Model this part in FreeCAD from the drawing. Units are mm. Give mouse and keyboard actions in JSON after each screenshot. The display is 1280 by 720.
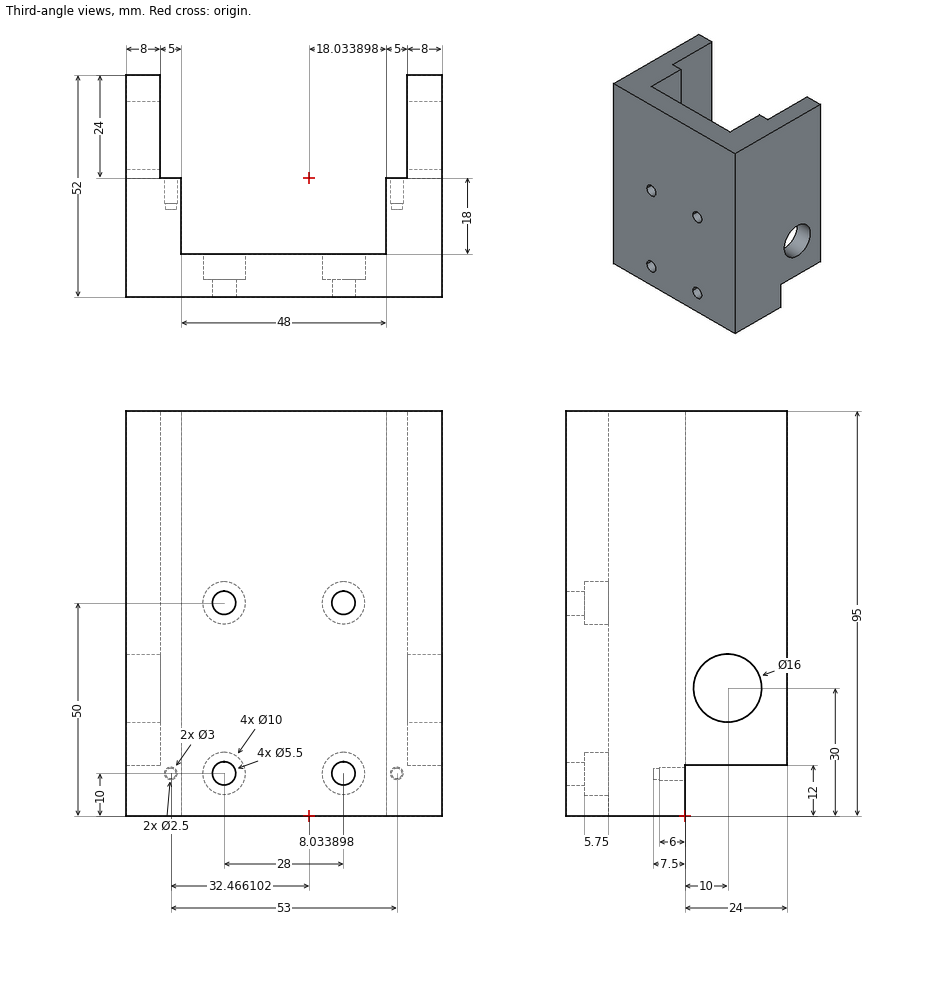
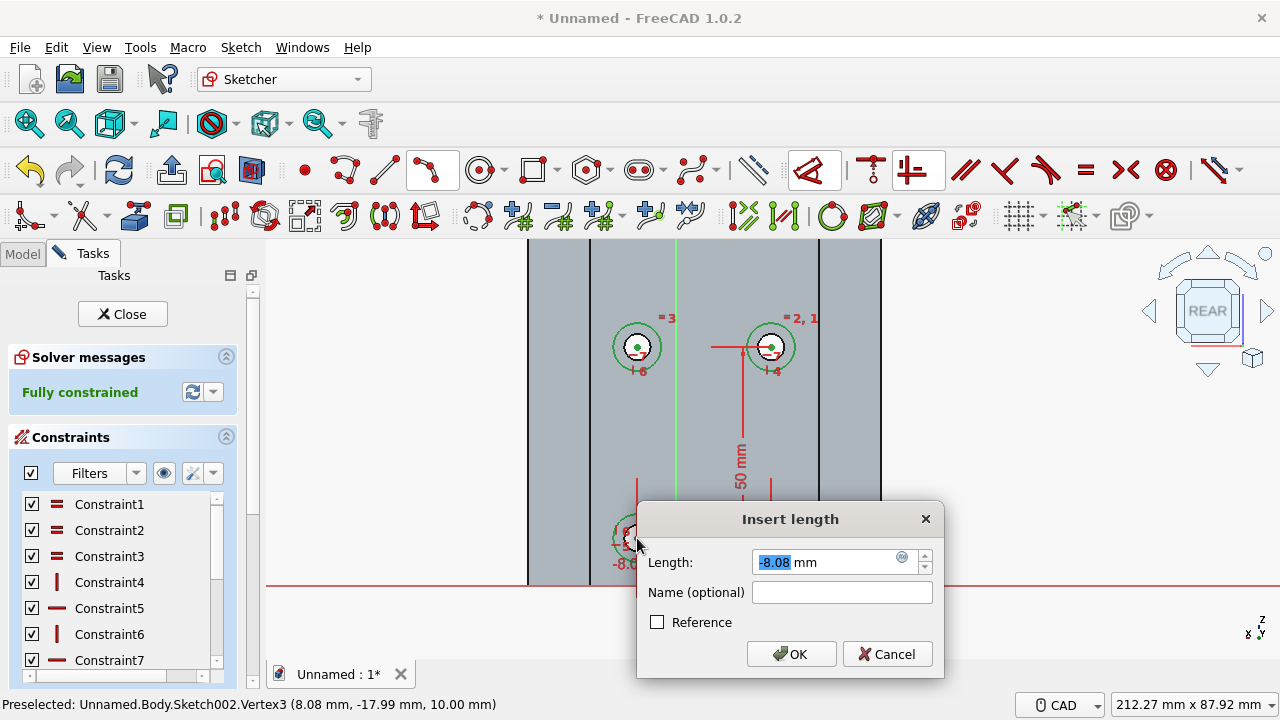
{"action": "type", "text": "-8.033898"}
{"action": "key", "text": "Return"}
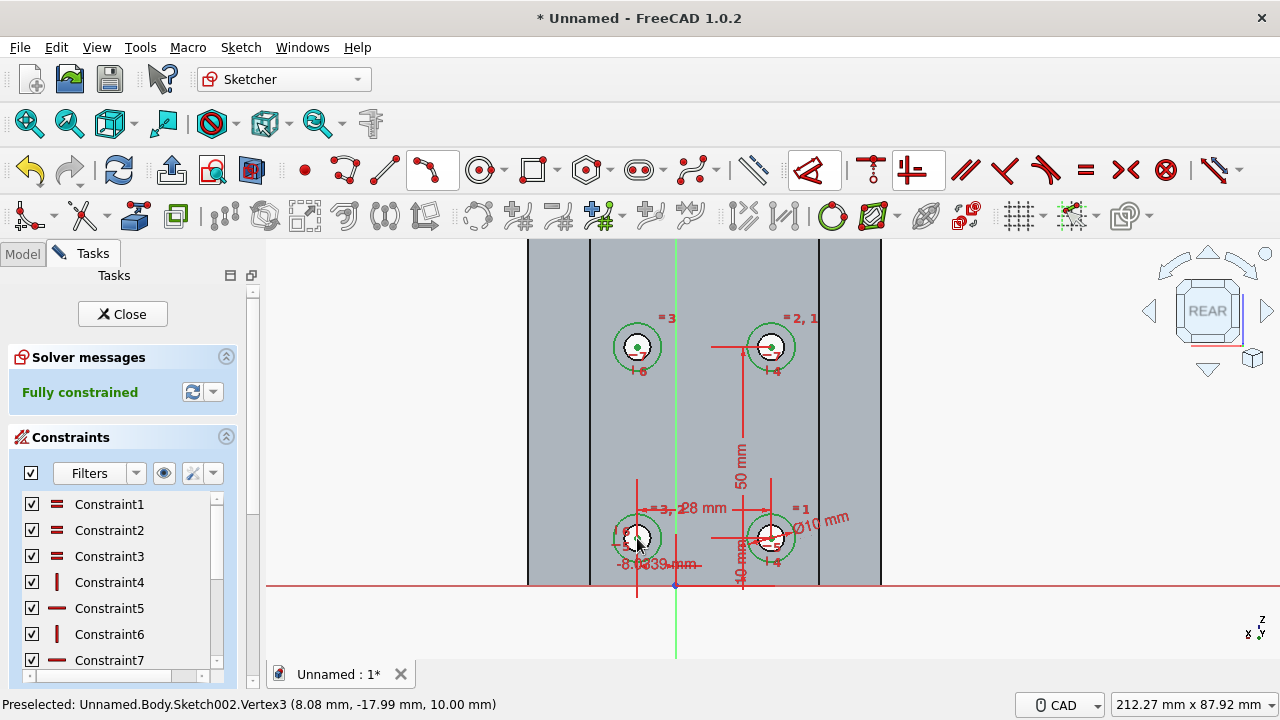
{"action": "left_click", "coordinate": [123, 314]}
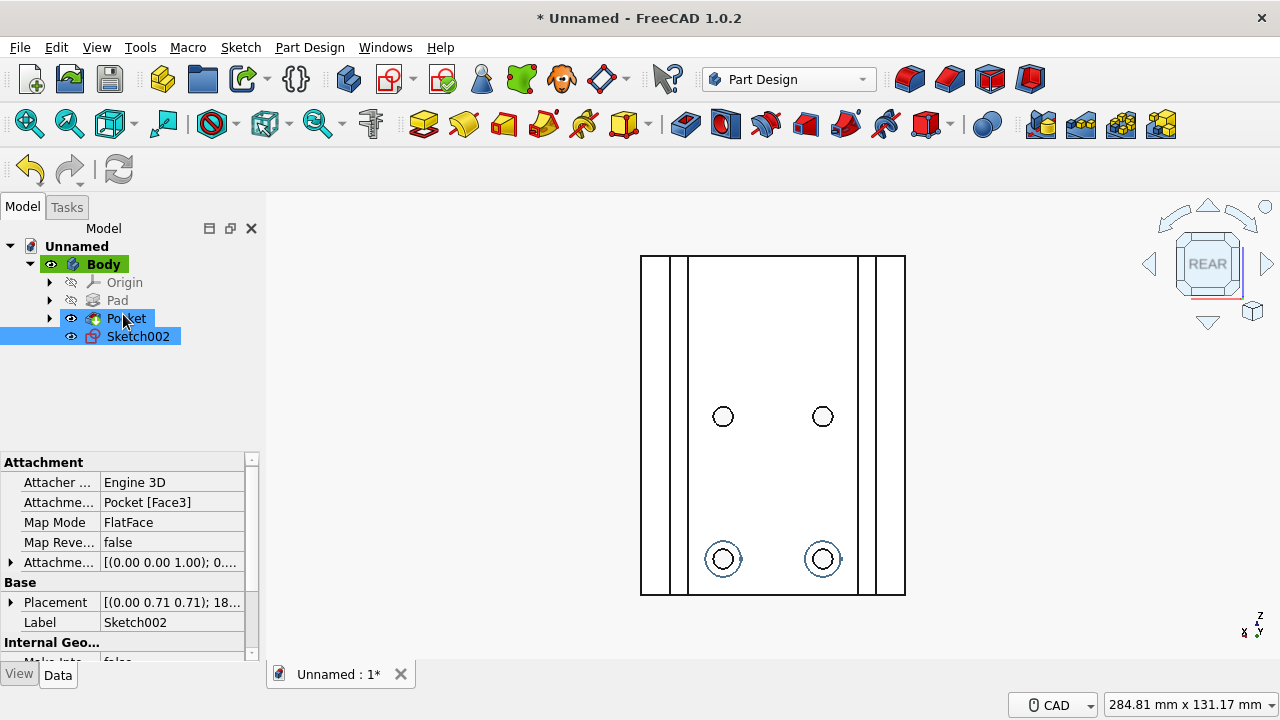
{"action": "left_click", "coordinate": [686, 124]}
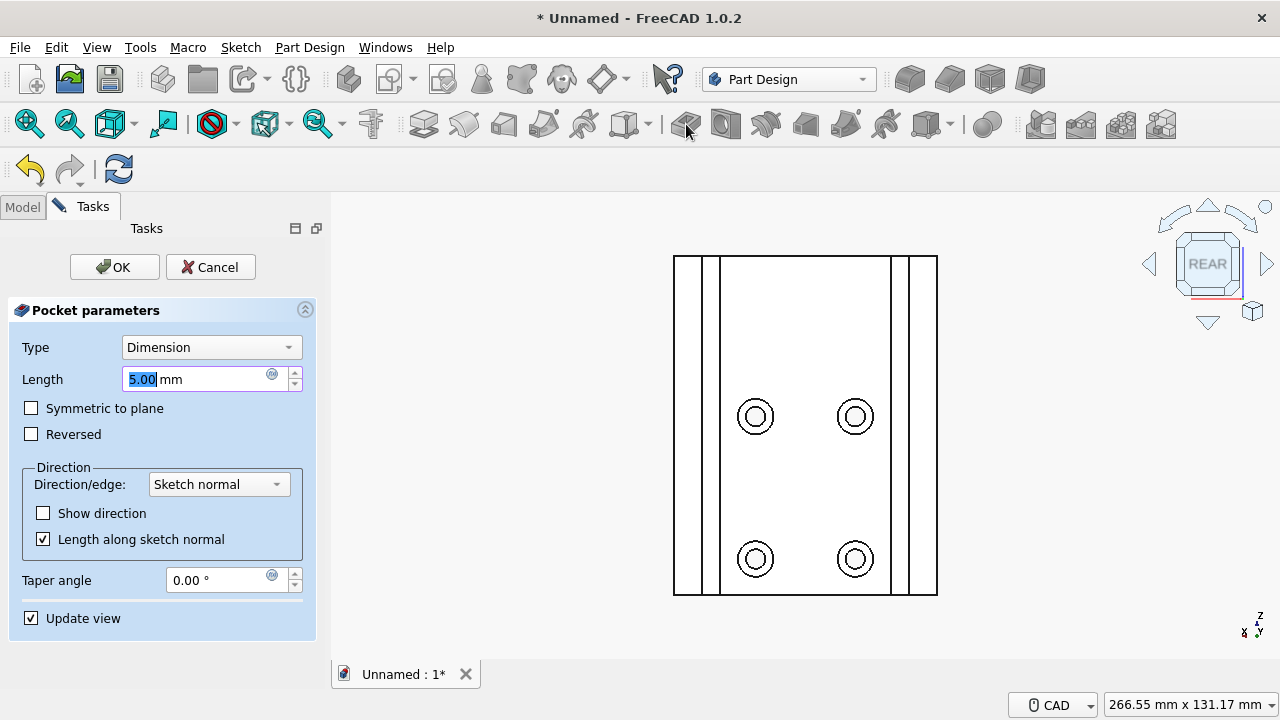
{"action": "type", "text": "5.75"}
{"action": "key", "text": "Tab"}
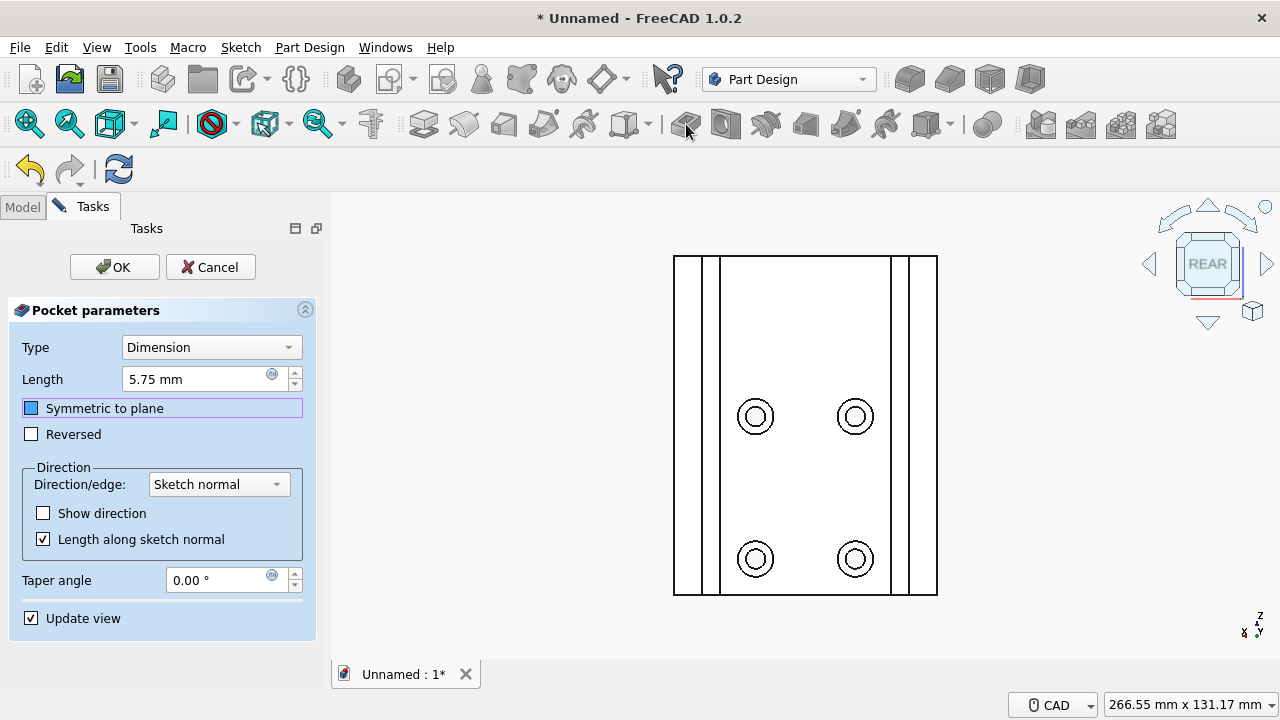
{"action": "left_click", "coordinate": [115, 267]}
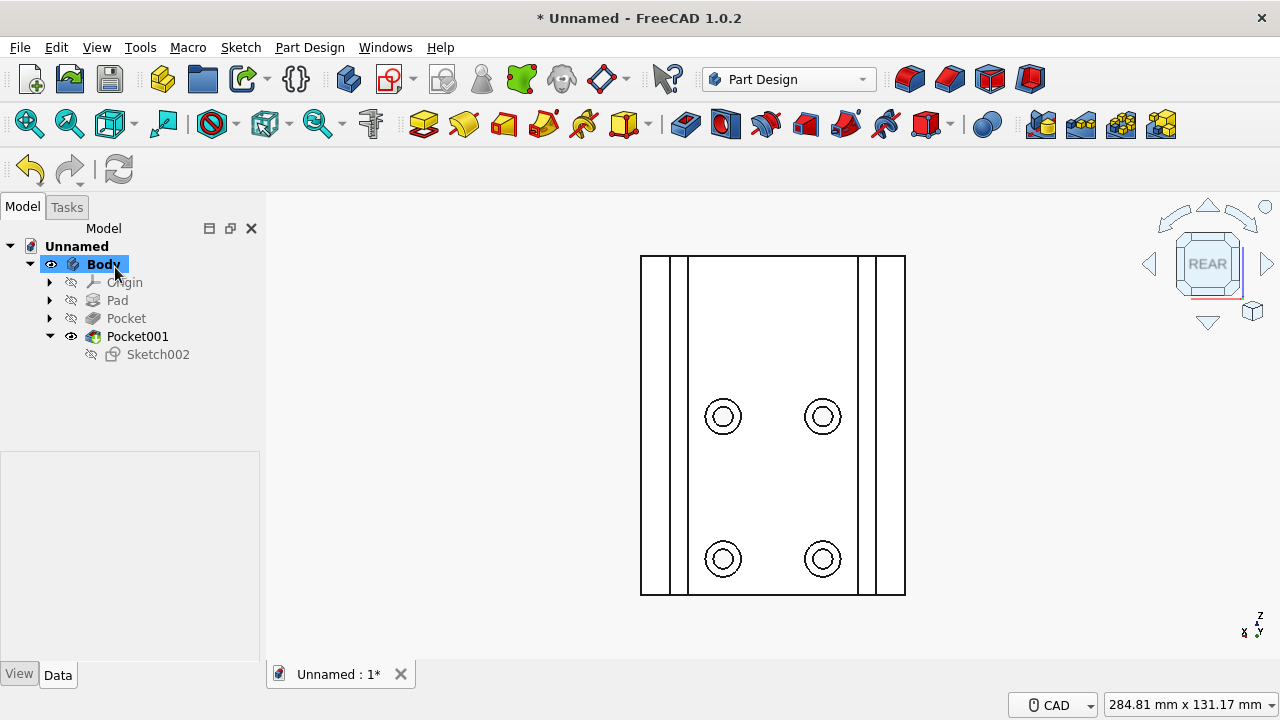
{"action": "key", "text": "6"}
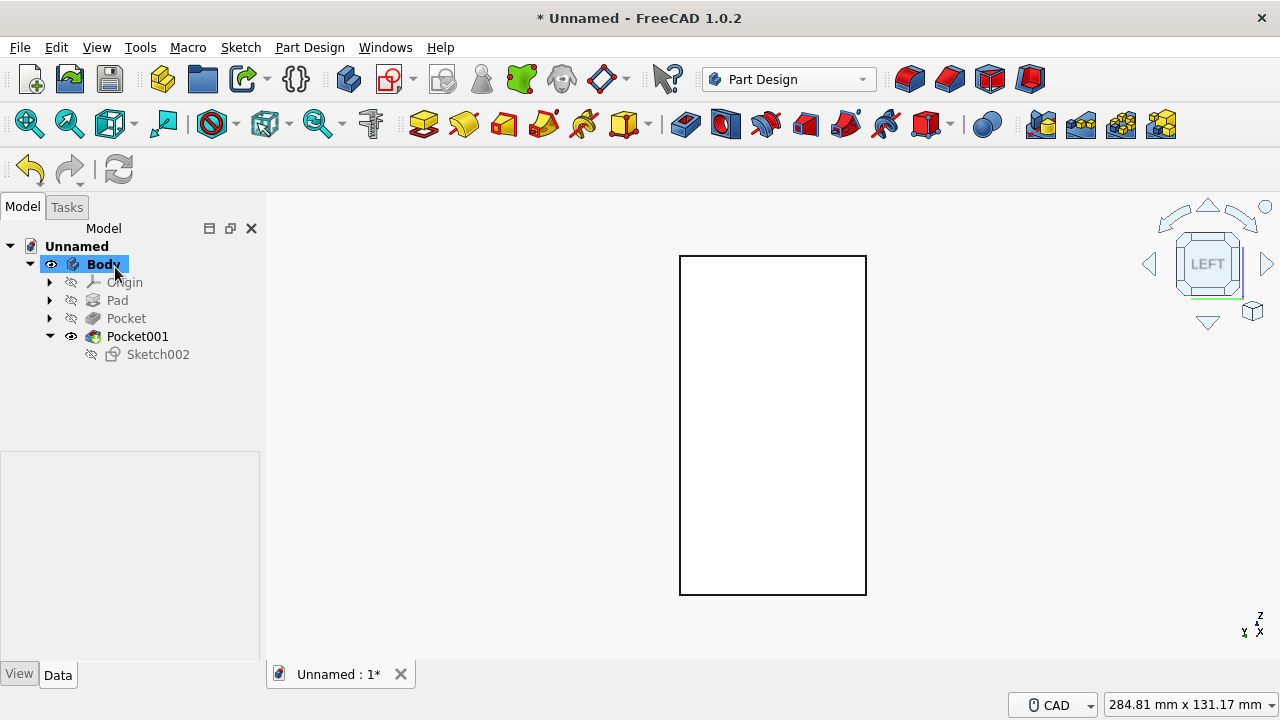
{"action": "left_click", "coordinate": [773, 376]}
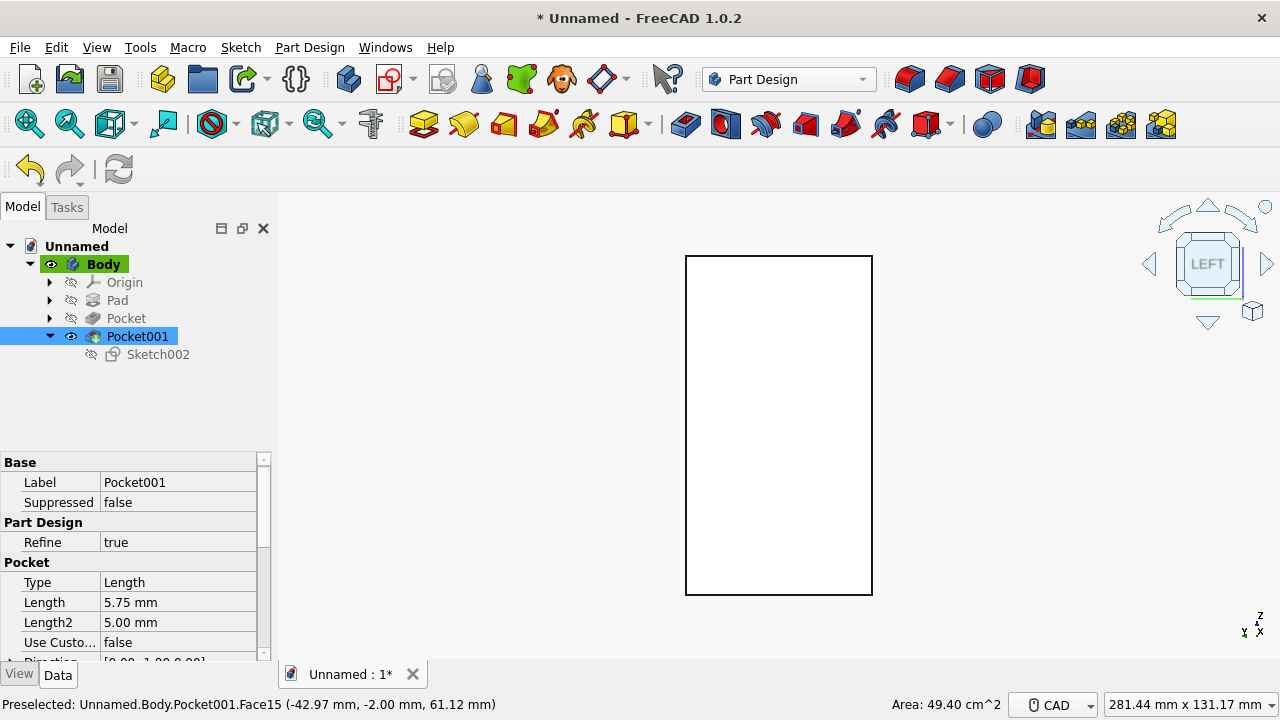
{"action": "left_click", "coordinate": [390, 80]}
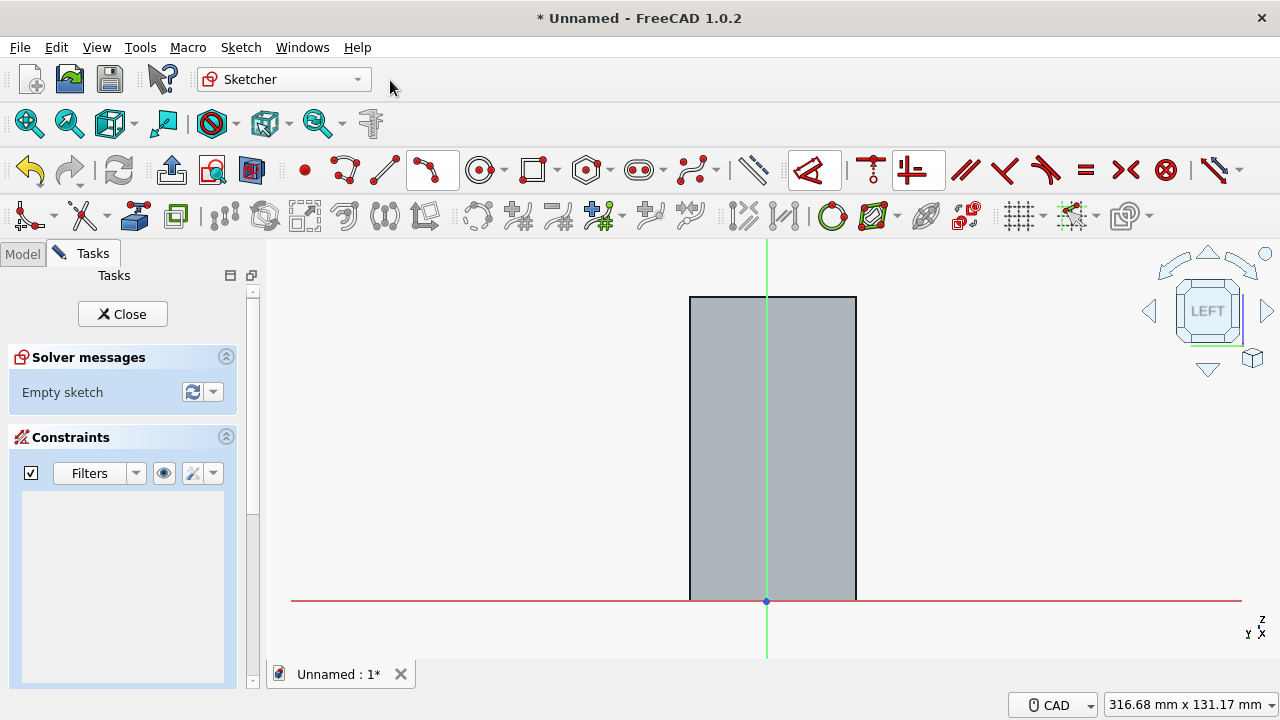
{"action": "scroll", "coordinate": [732, 603], "scroll_direction": "up", "scroll_amount": 10}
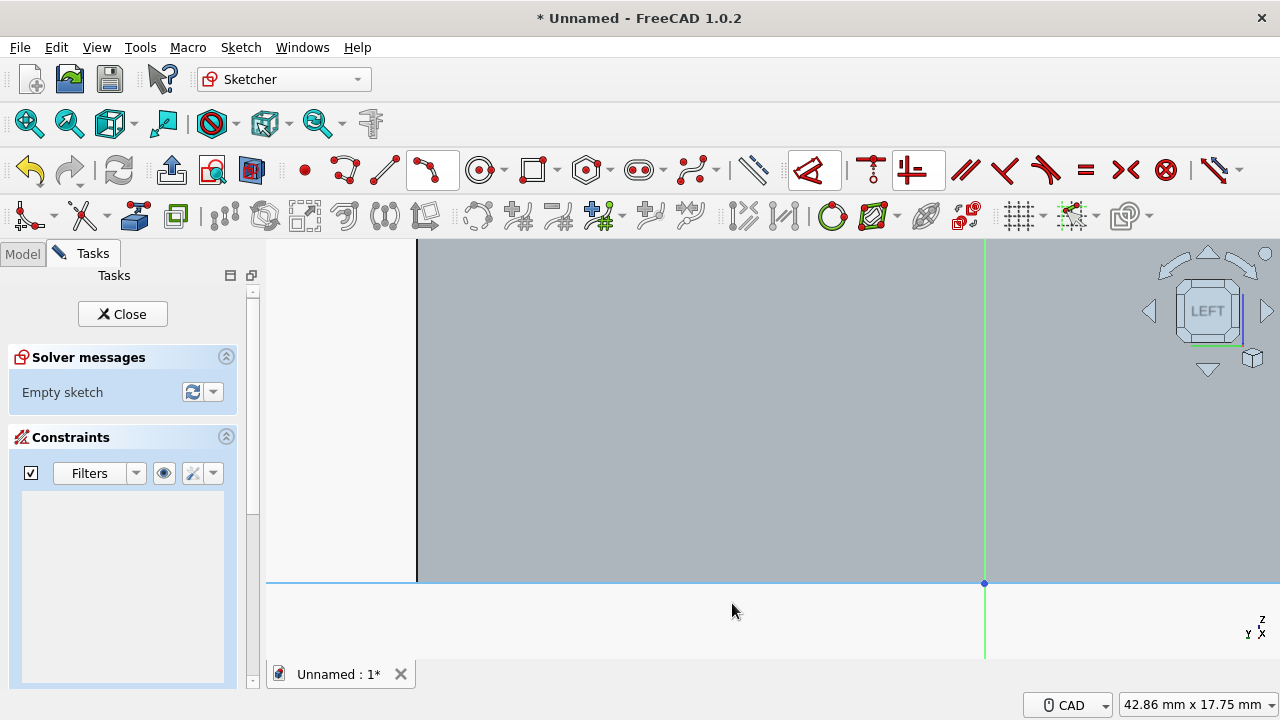
{"action": "key", "text": "g r"}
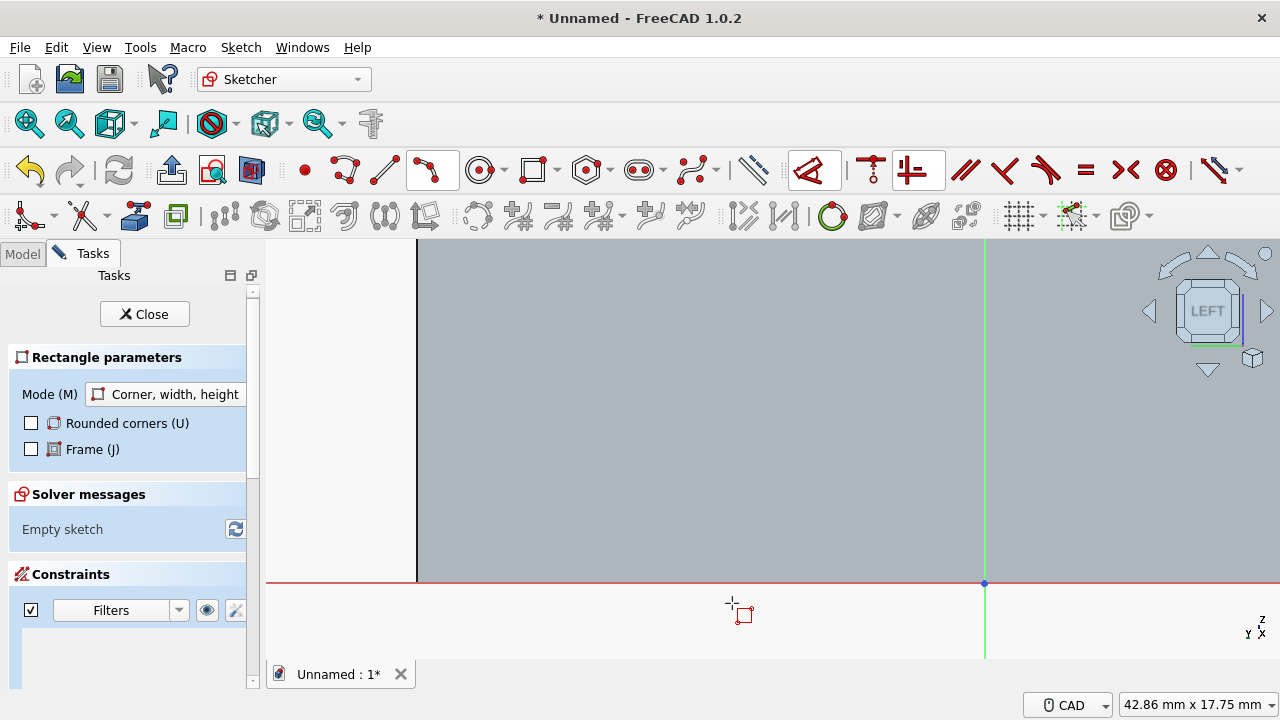
{"action": "left_click", "coordinate": [985, 583]}
{"action": "left_click", "coordinate": [417, 299]}
{"action": "key", "text": "Escape"}